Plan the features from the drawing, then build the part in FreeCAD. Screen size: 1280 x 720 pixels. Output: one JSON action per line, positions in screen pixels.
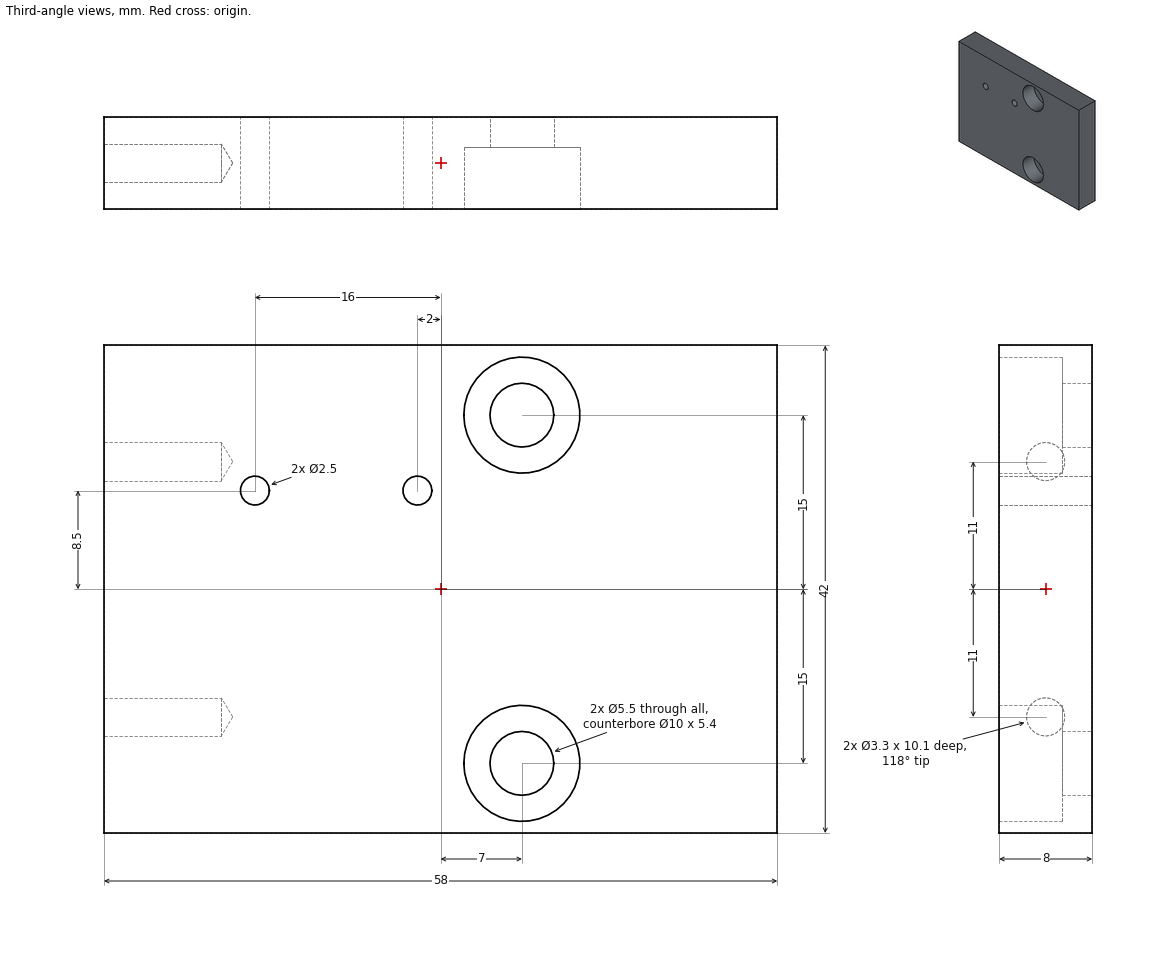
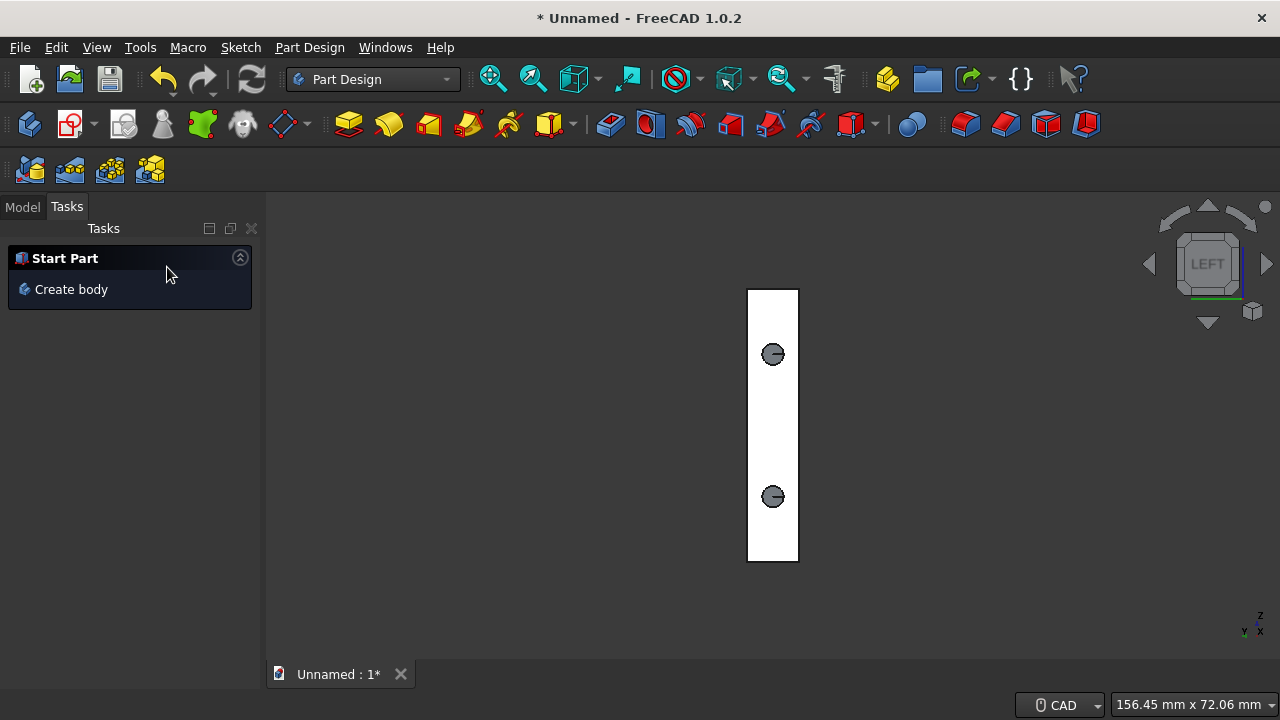
{"action": "key", "text": "0"}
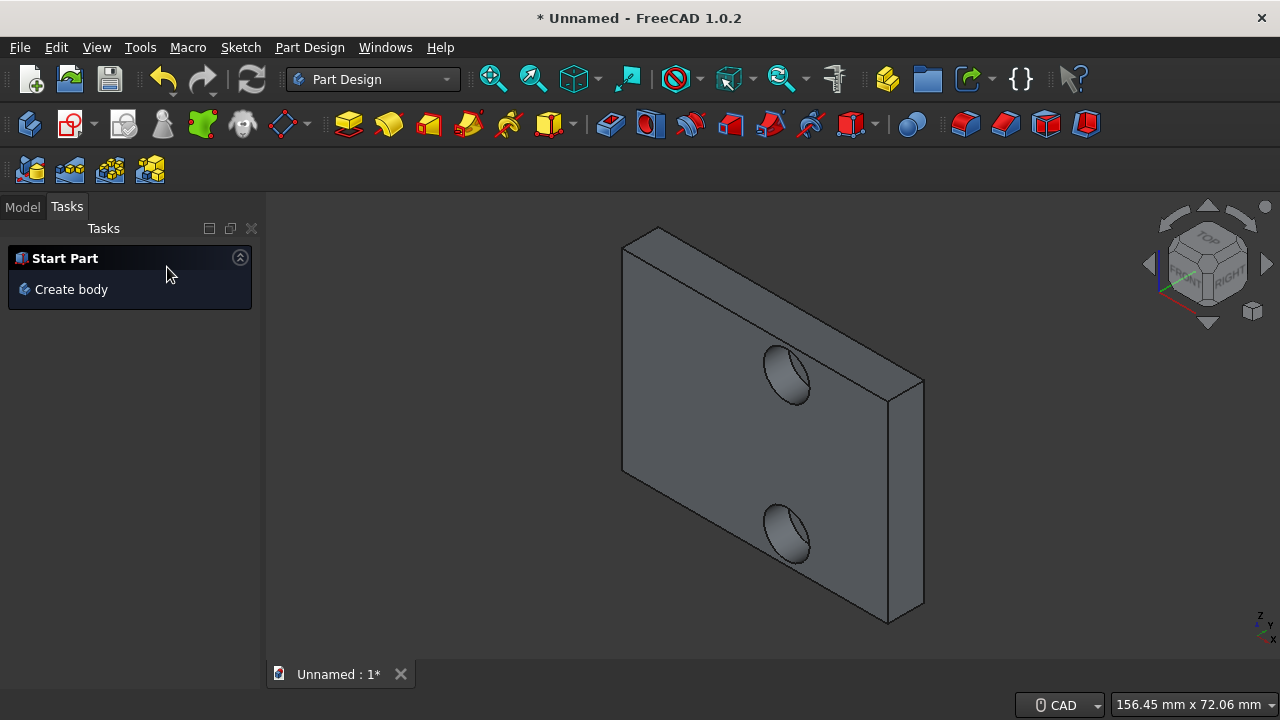
{"action": "left_click", "coordinate": [717, 413]}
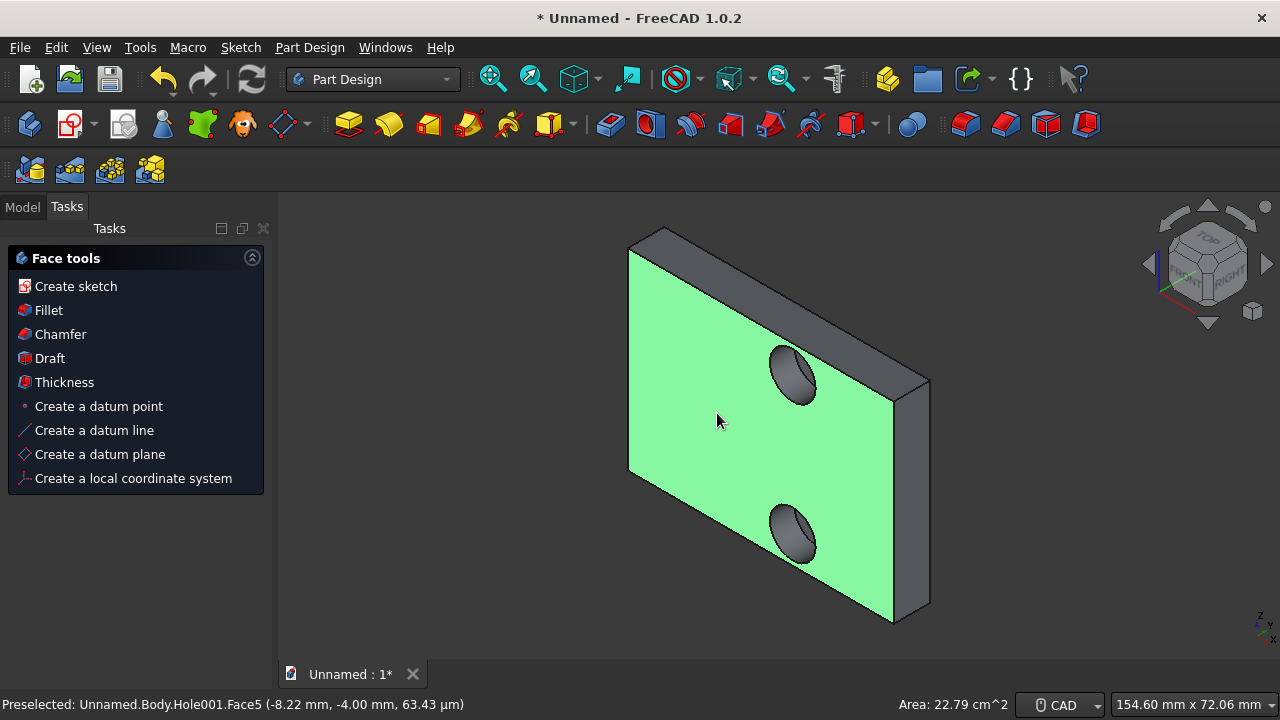
{"action": "left_click", "coordinate": [70, 124]}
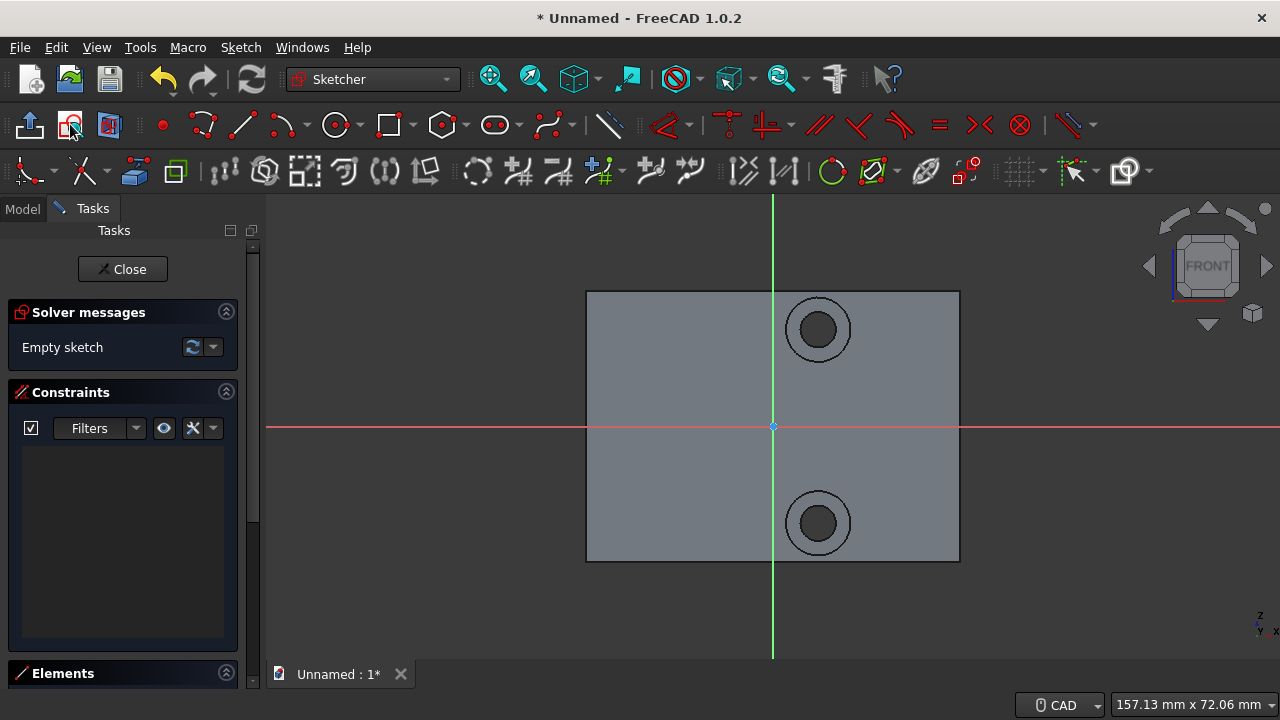
{"action": "scroll", "coordinate": [721, 387], "scroll_direction": "up", "scroll_amount": 8}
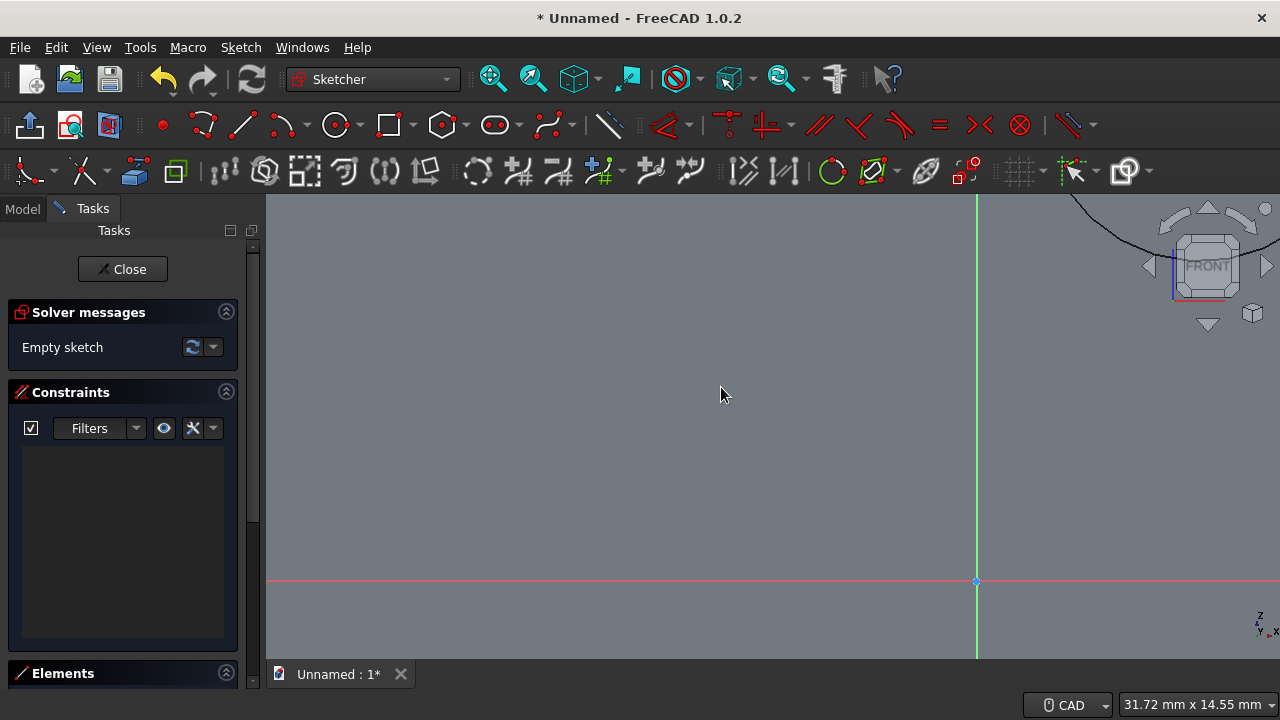
{"action": "key", "text": "g c"}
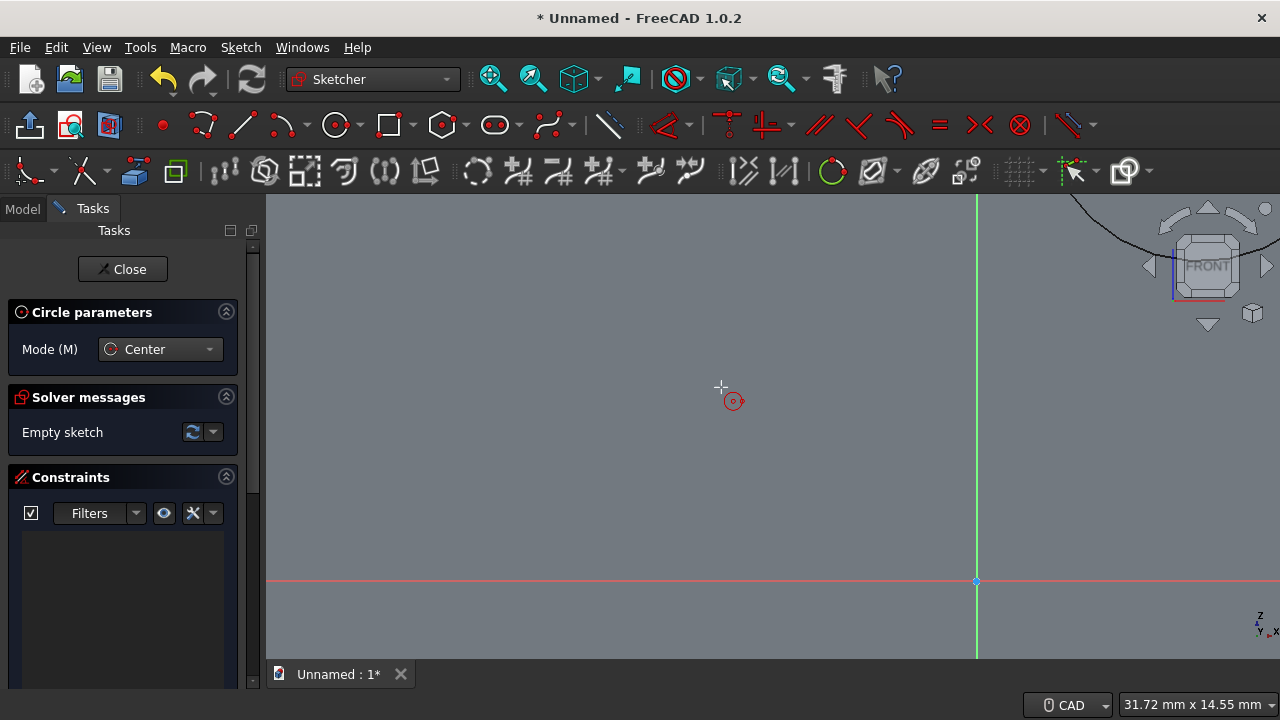
{"action": "left_click", "coordinate": [465, 309]}
{"action": "left_click", "coordinate": [494, 281]}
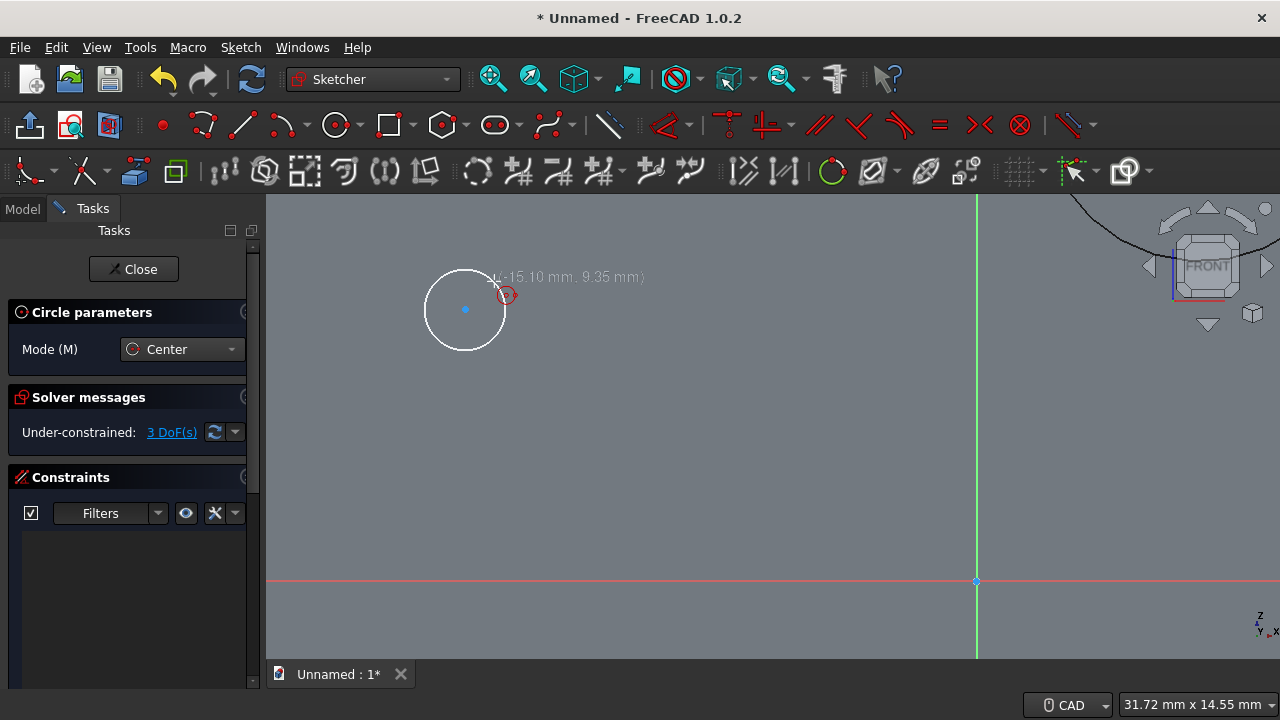
{"action": "left_click", "coordinate": [913, 309]}
{"action": "left_click", "coordinate": [941, 281]}
{"action": "key", "text": "Escape"}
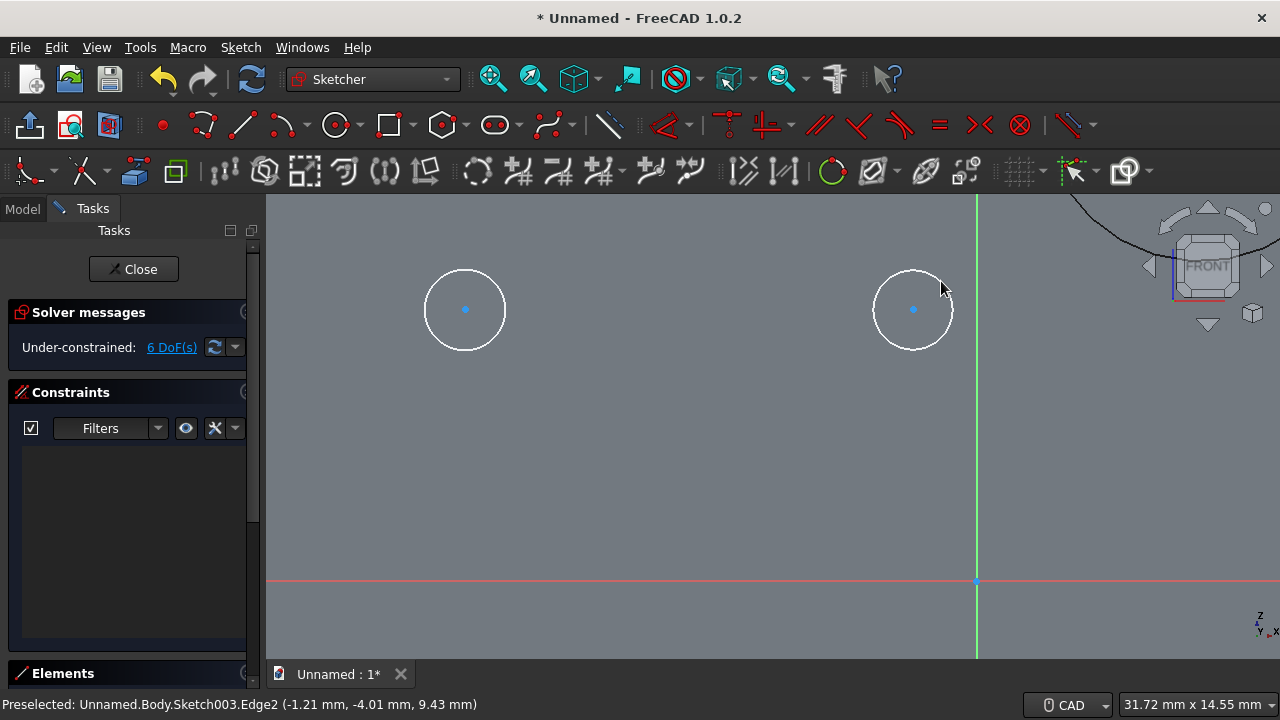
{"action": "left_click", "coordinate": [493, 281]}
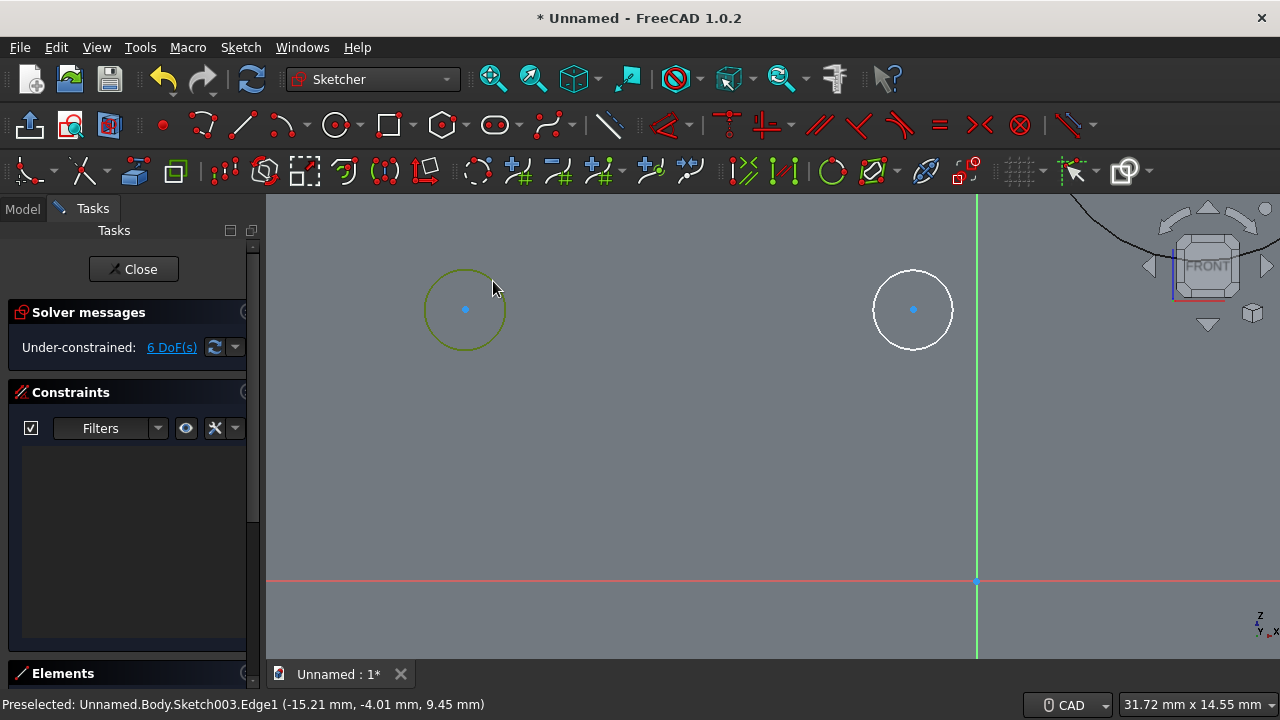
{"action": "left_click", "coordinate": [941, 282]}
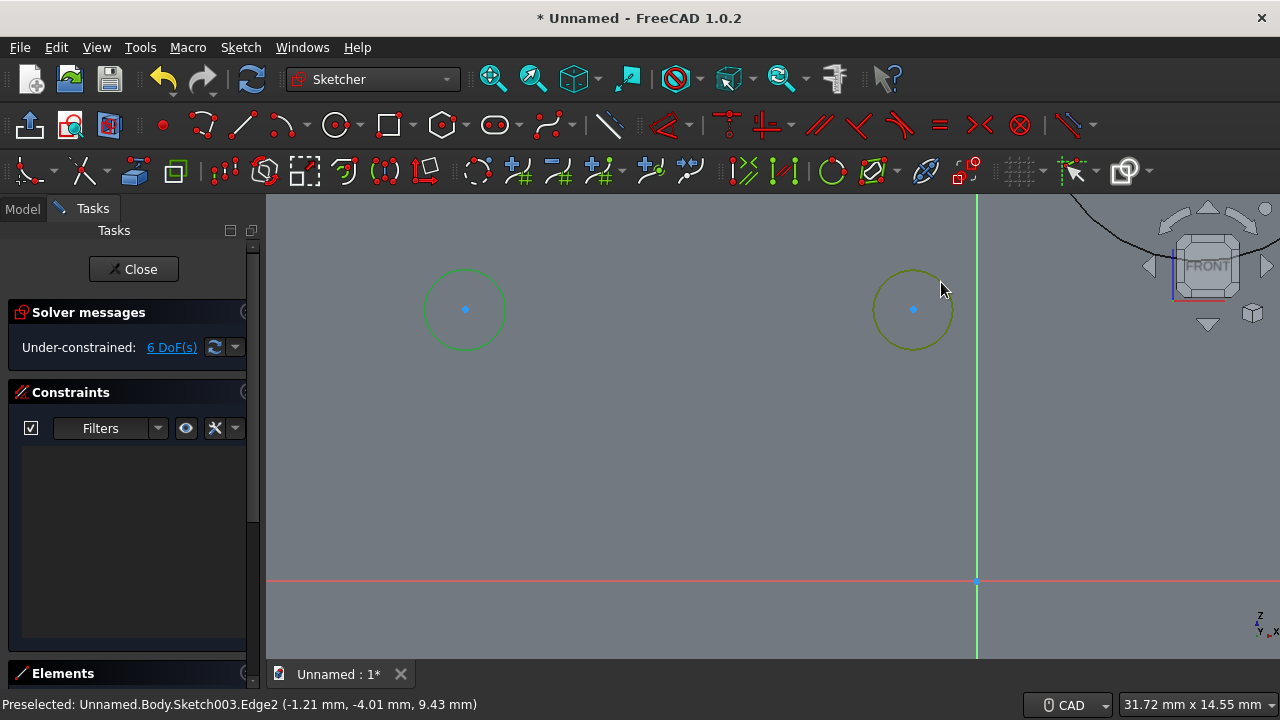
{"action": "left_click", "coordinate": [940, 126]}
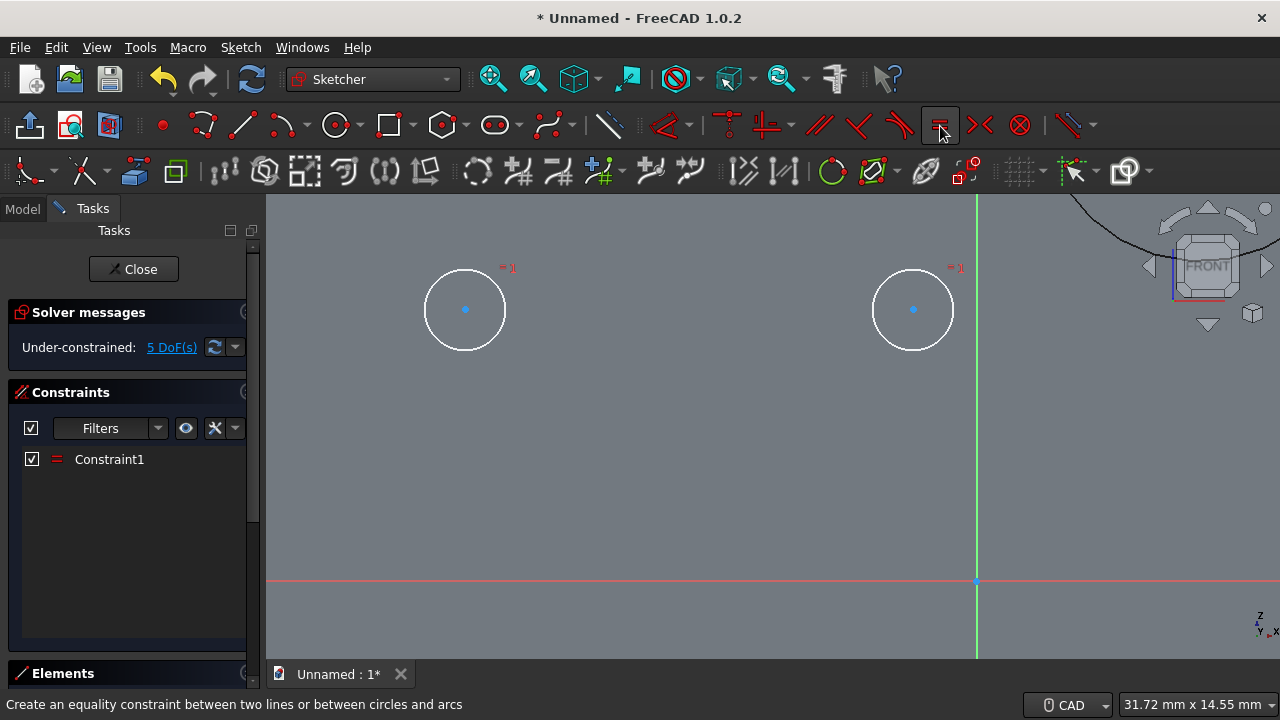
{"action": "left_click", "coordinate": [465, 310]}